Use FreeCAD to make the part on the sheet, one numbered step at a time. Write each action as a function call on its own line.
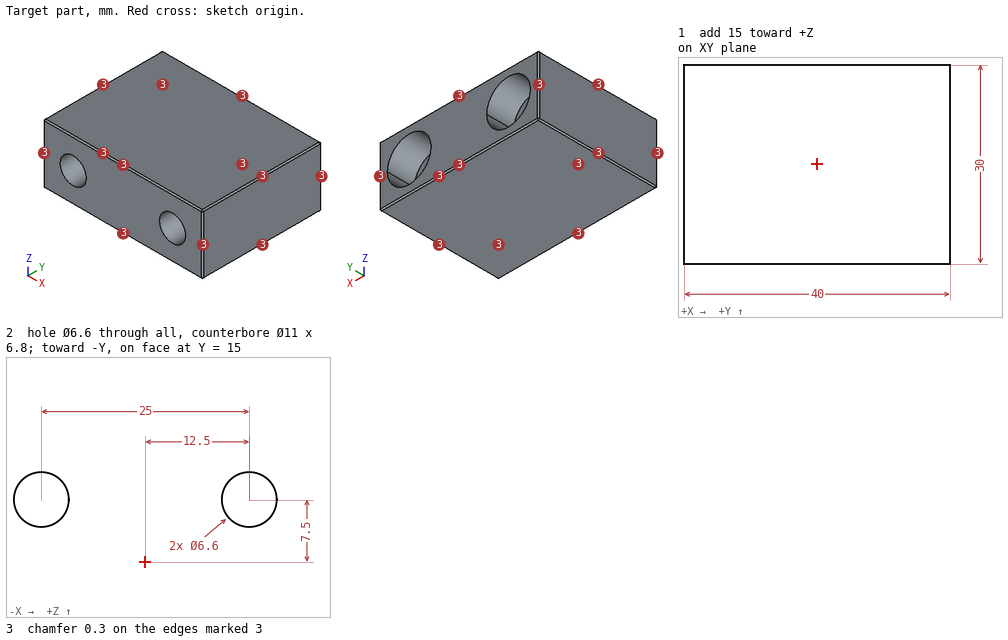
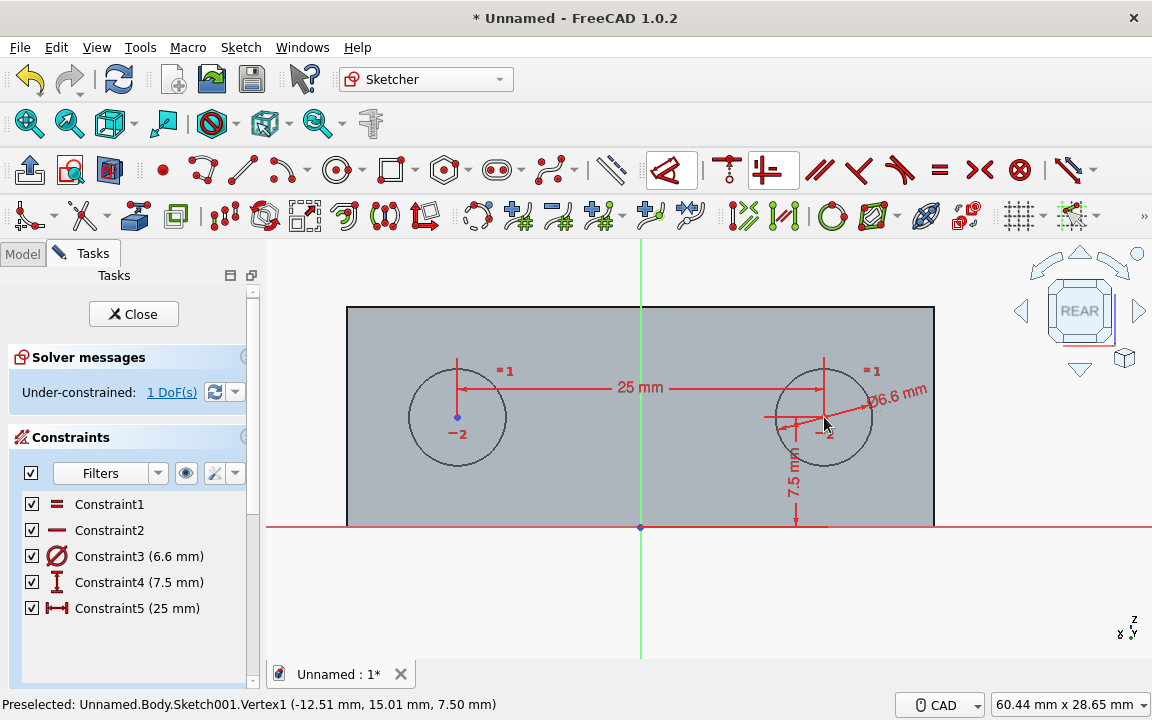
click(692, 170)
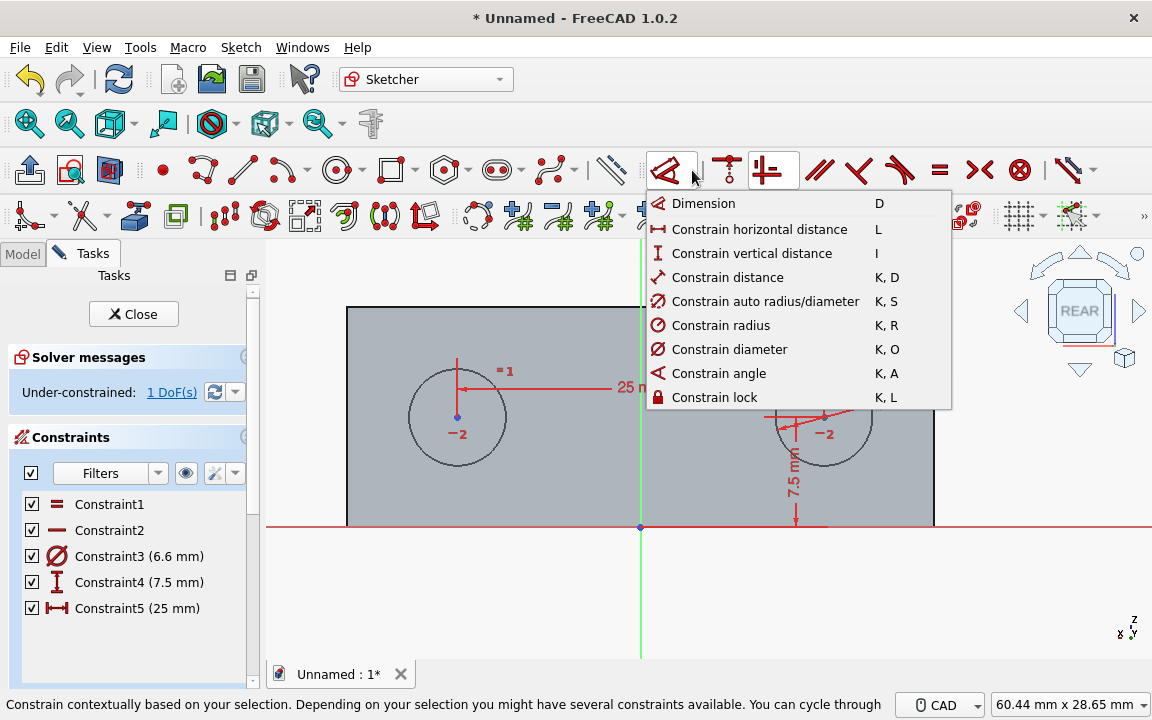
click(799, 229)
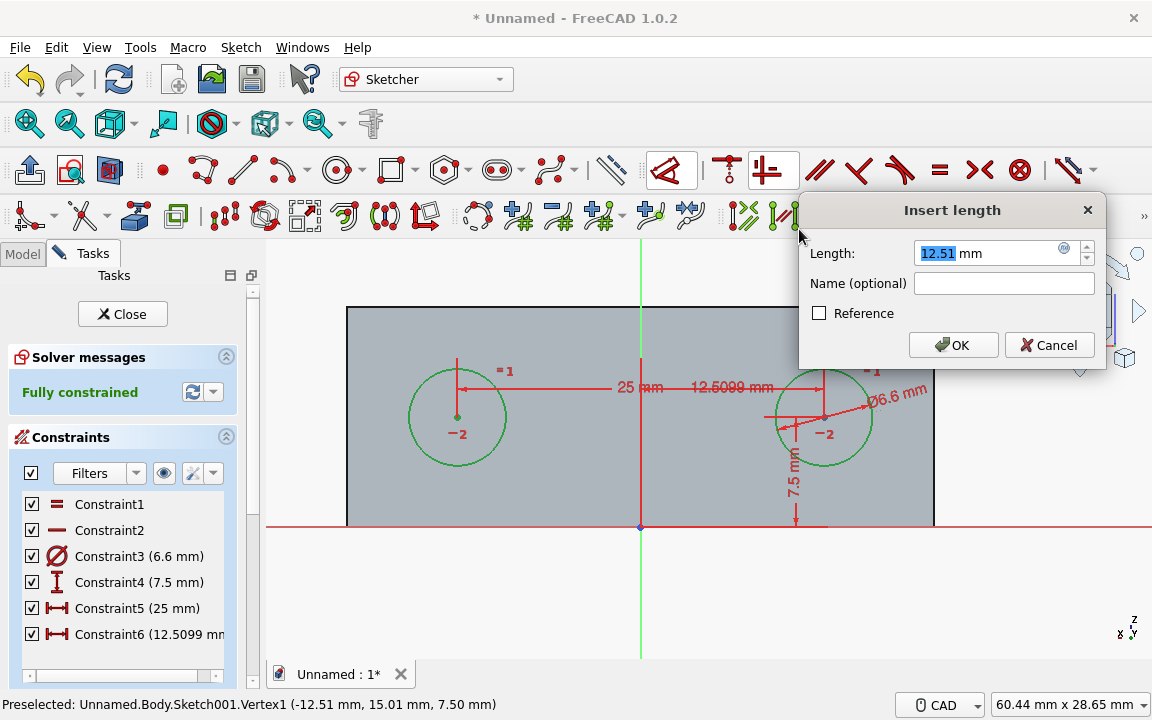
text(12.5)
key(Return)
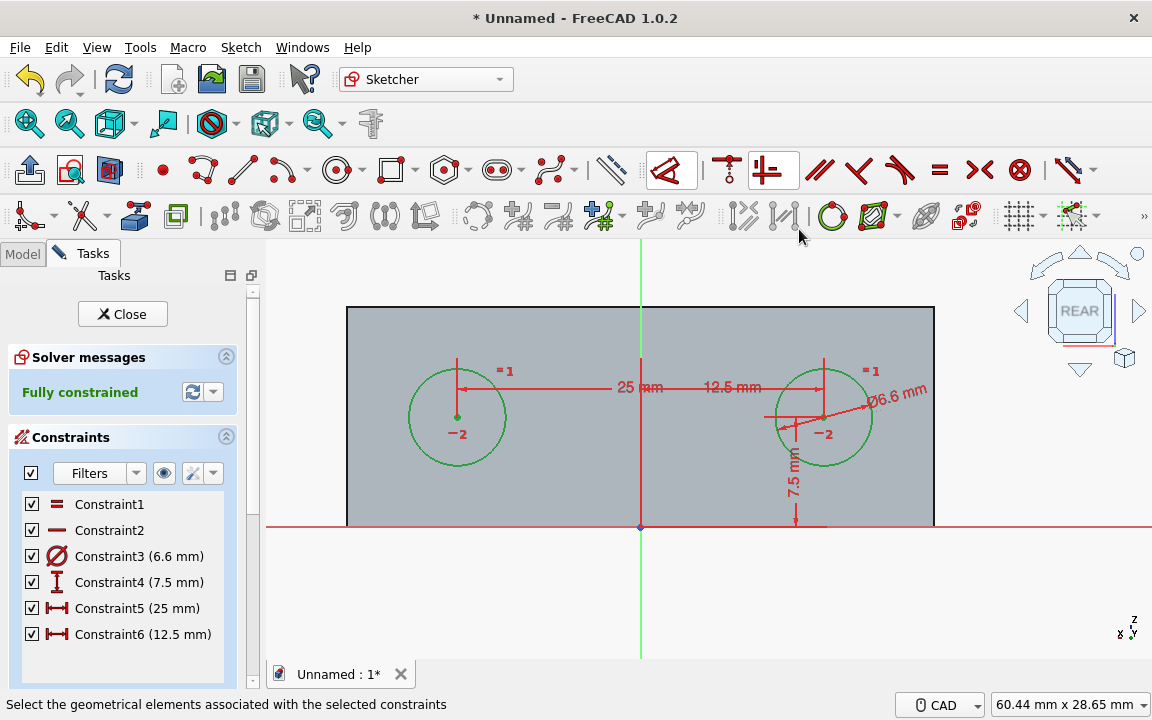
click(123, 314)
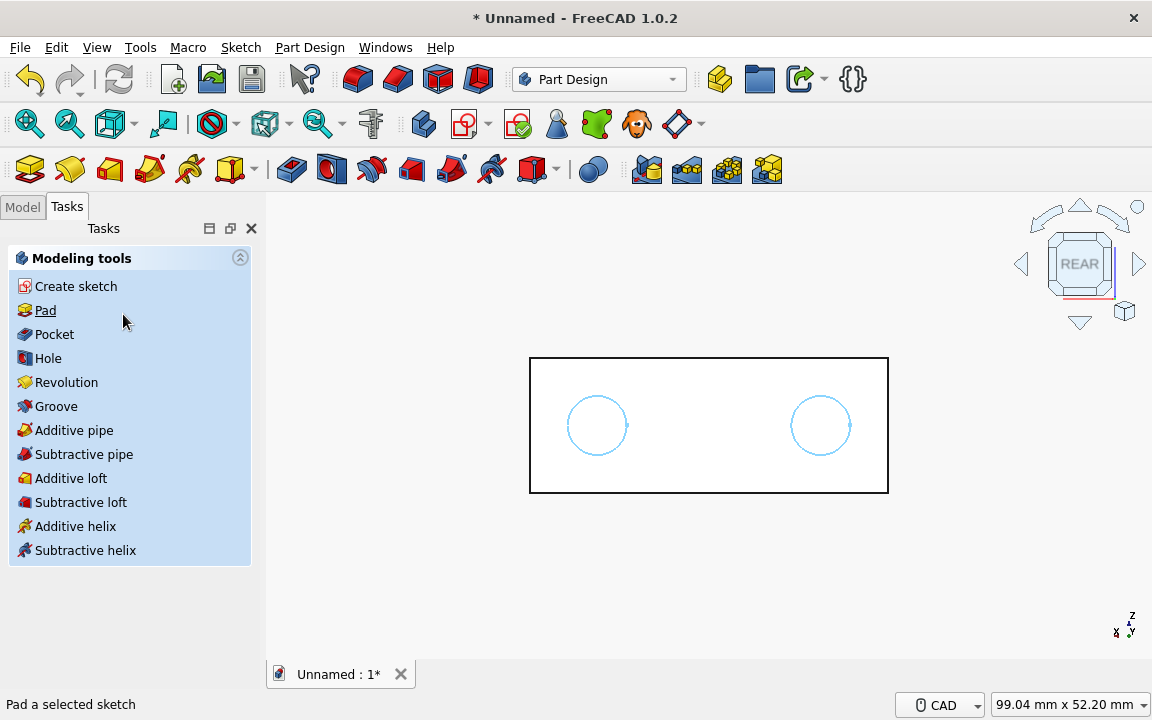
click(332, 170)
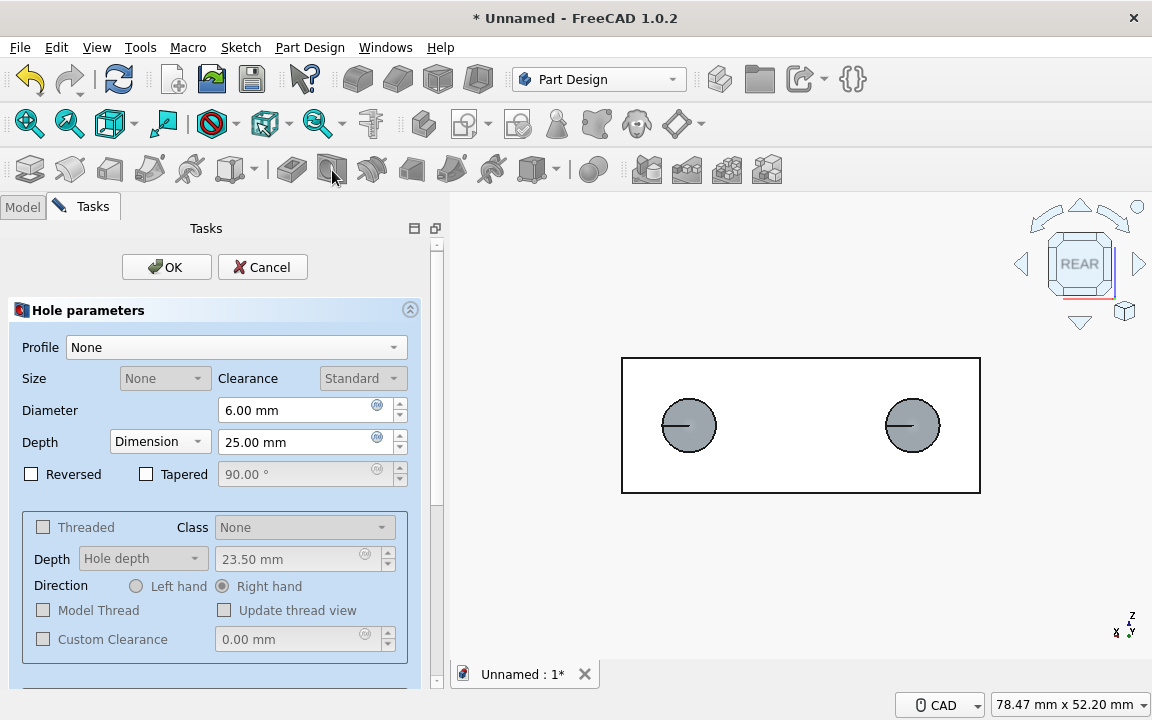
triple_click(305, 410)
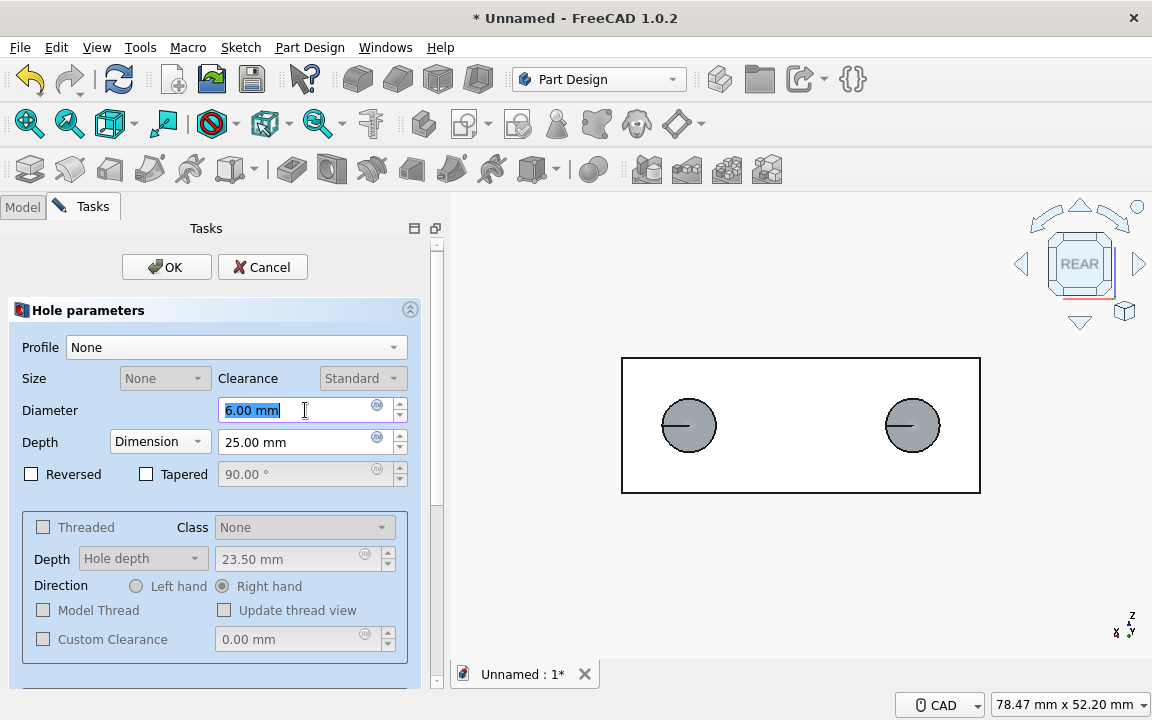
text(6.6)
key(Tab)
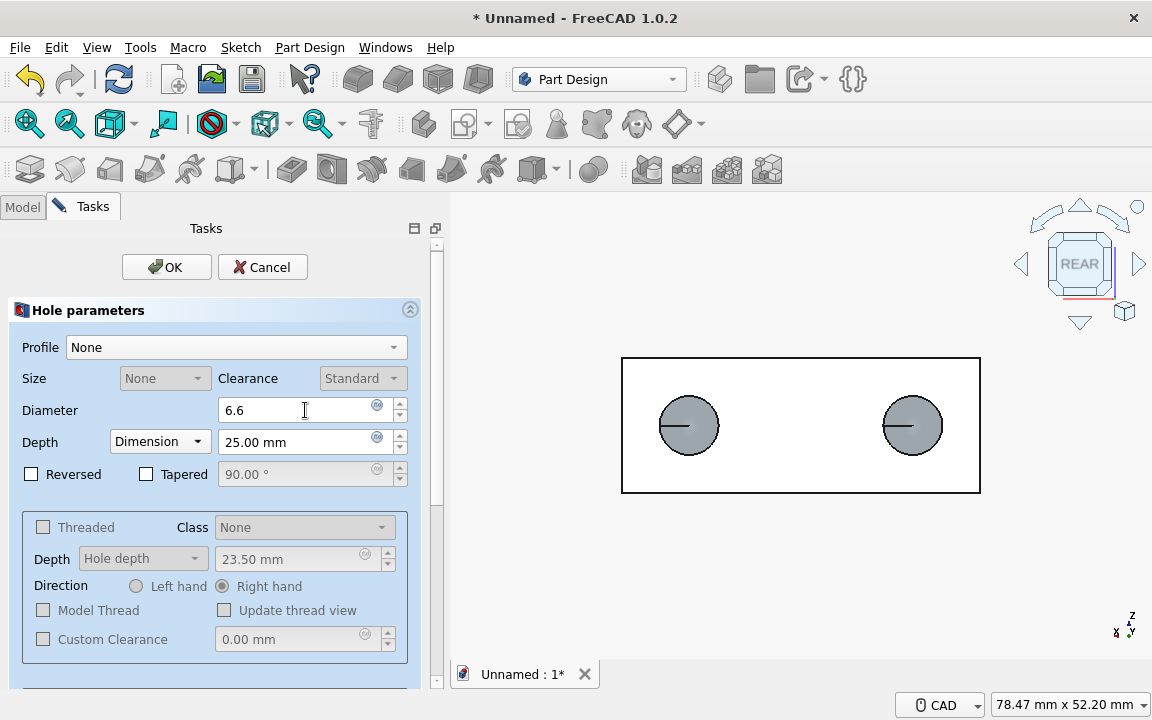
click(161, 442)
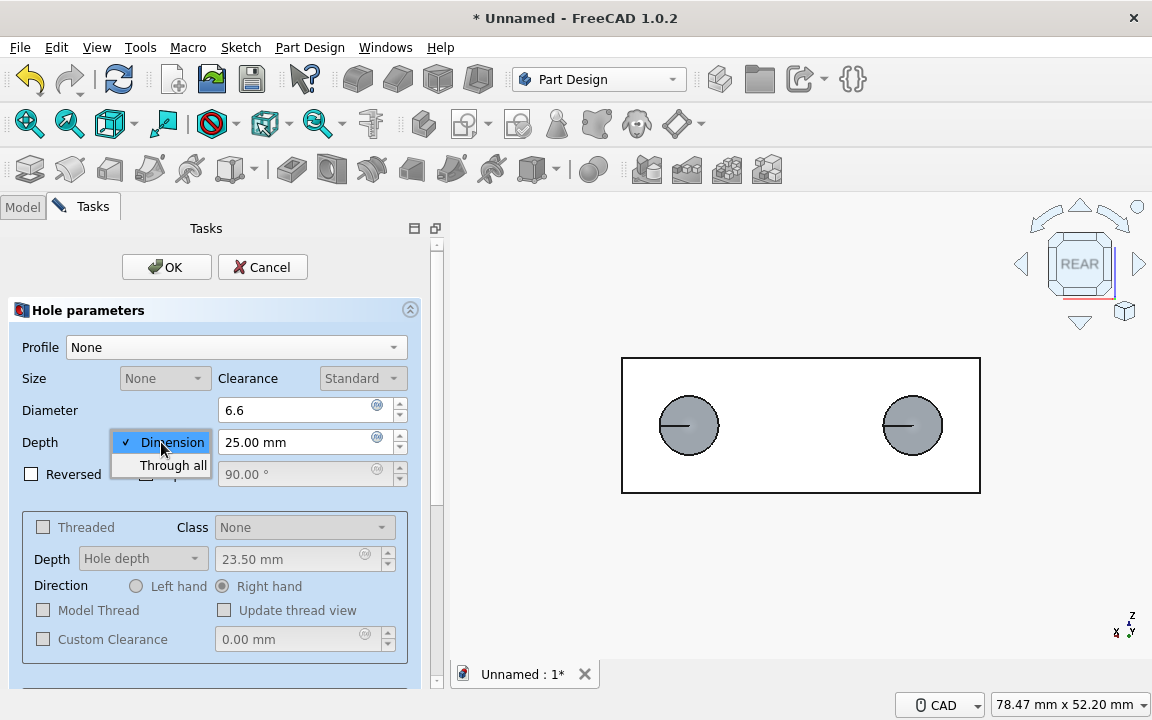
click(160, 466)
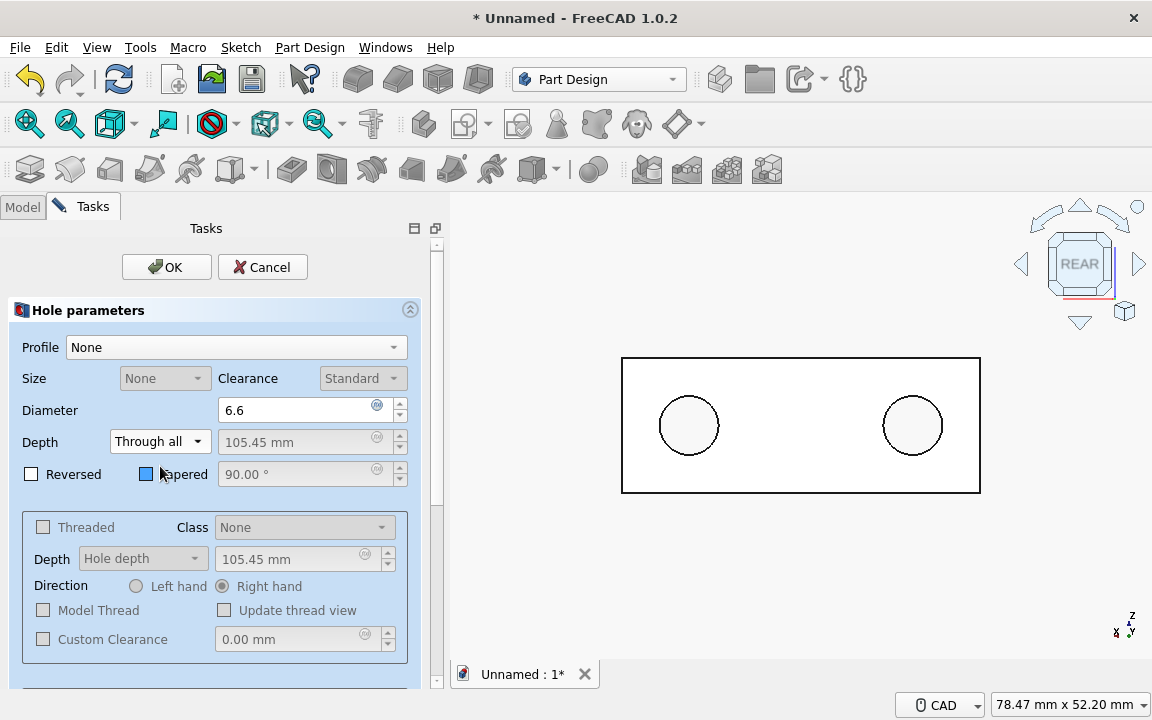
scroll(437, 463, down, 2)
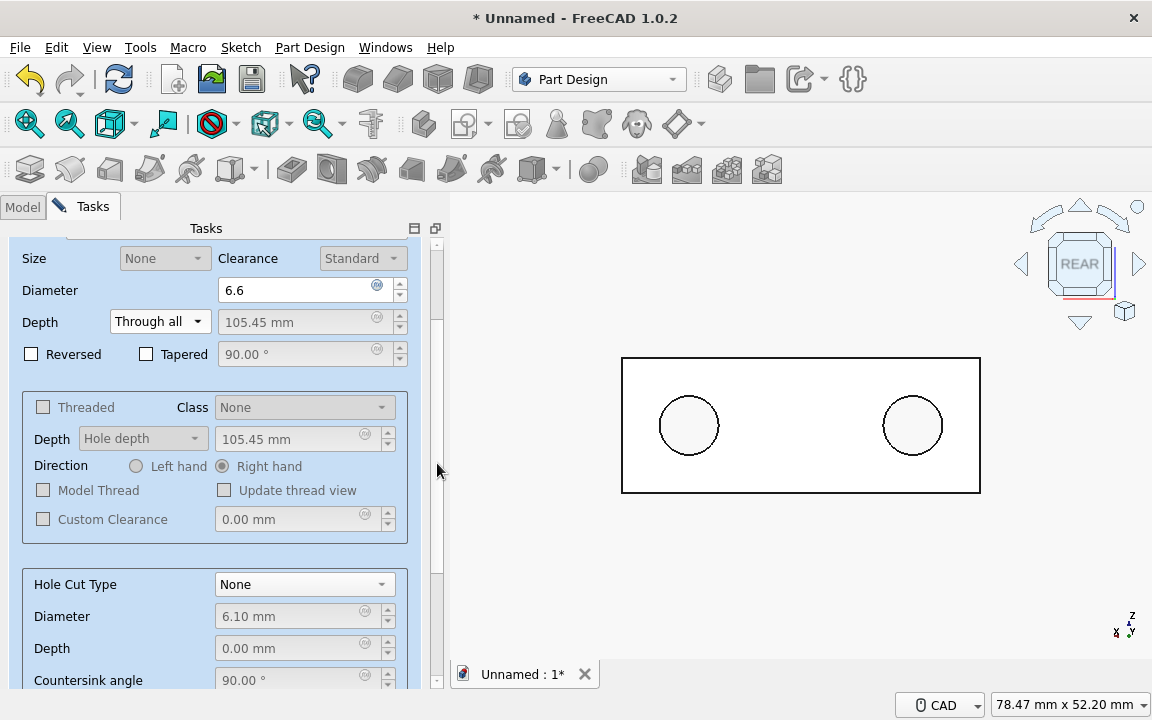
click(306, 584)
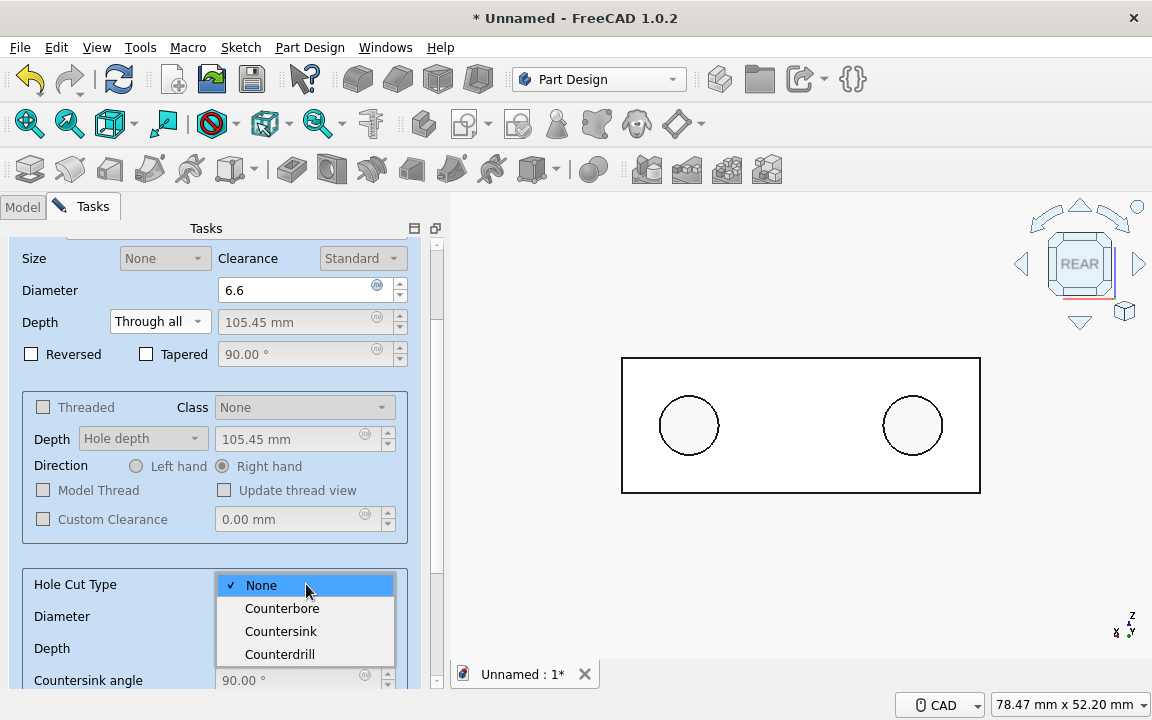
click(304, 608)